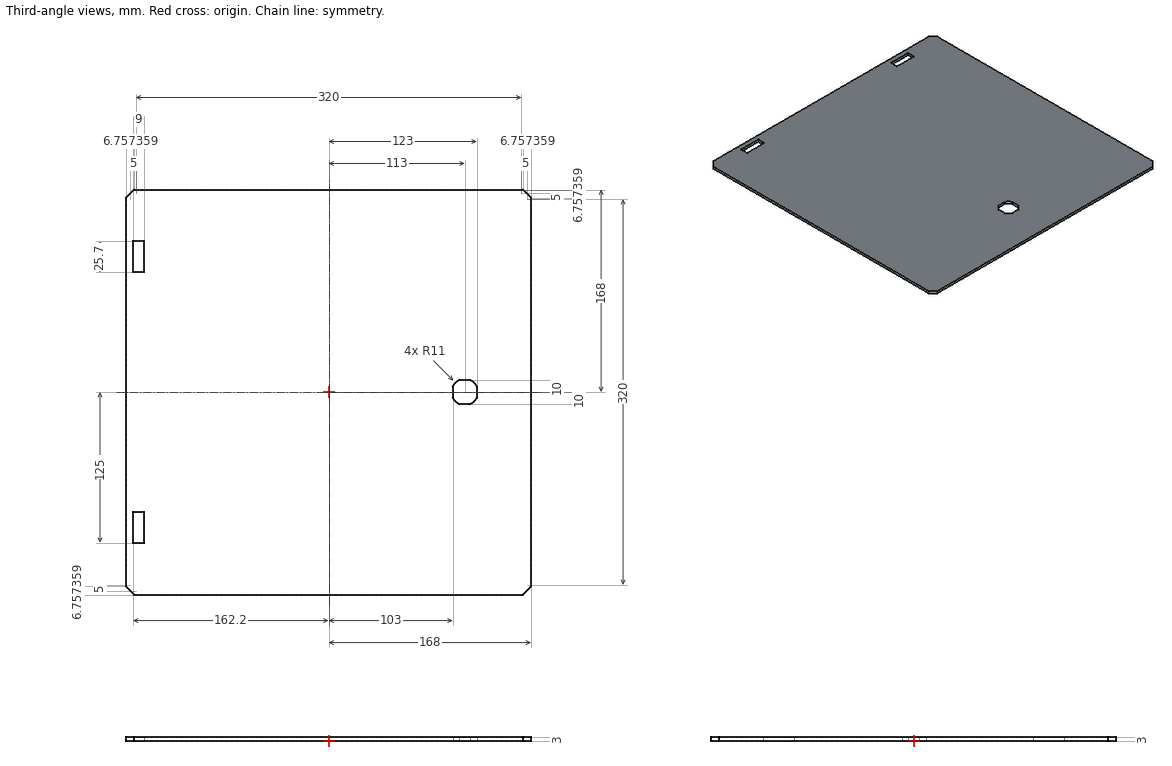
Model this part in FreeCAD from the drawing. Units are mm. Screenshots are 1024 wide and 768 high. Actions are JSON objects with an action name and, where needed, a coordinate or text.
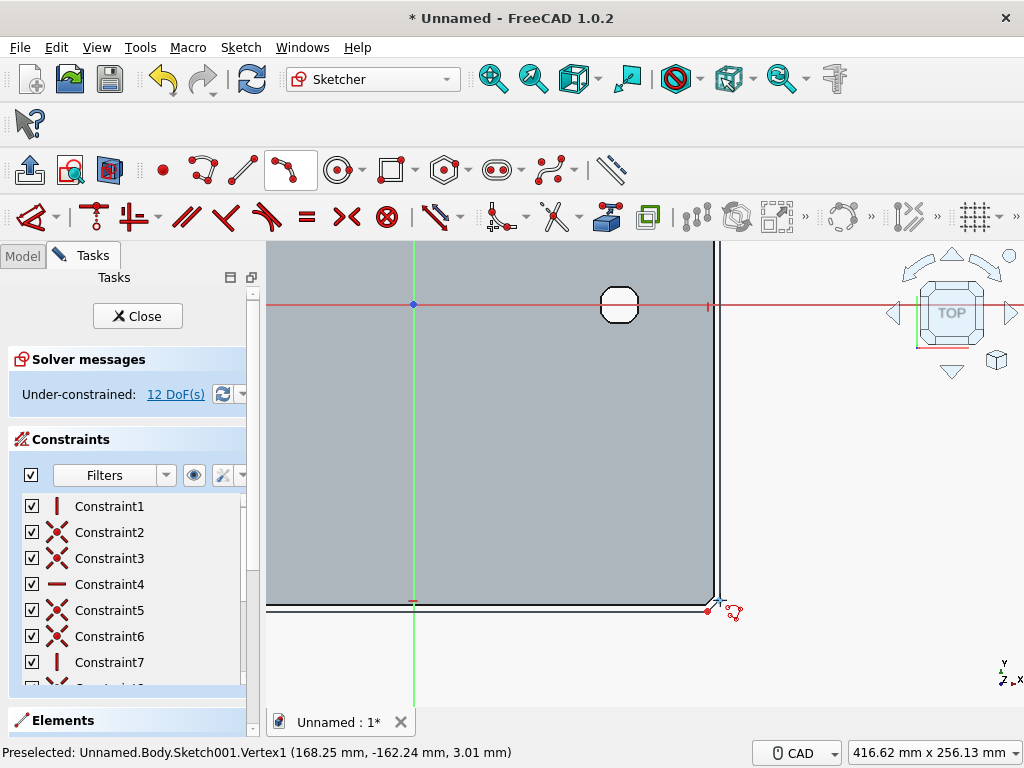
{"action": "scroll", "coordinate": [714, 596], "scroll_direction": "up", "scroll_amount": 6}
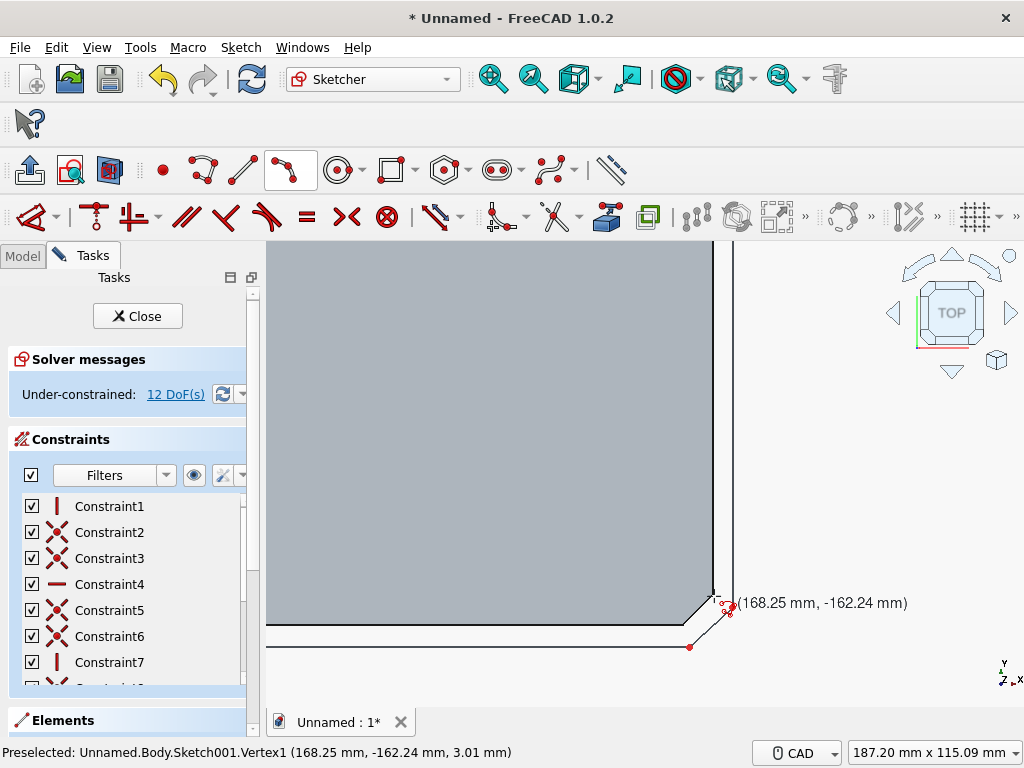
{"action": "left_click", "coordinate": [713, 594]}
{"action": "left_click", "coordinate": [683, 625]}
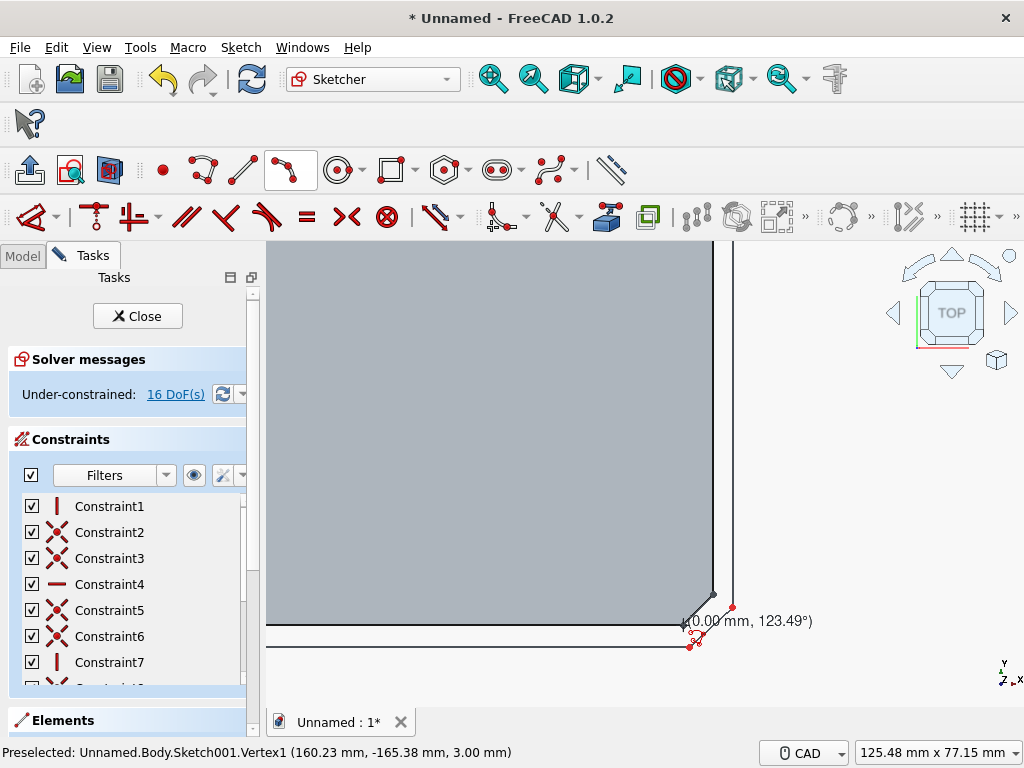
{"action": "scroll", "coordinate": [711, 606], "scroll_direction": "down", "scroll_amount": 10}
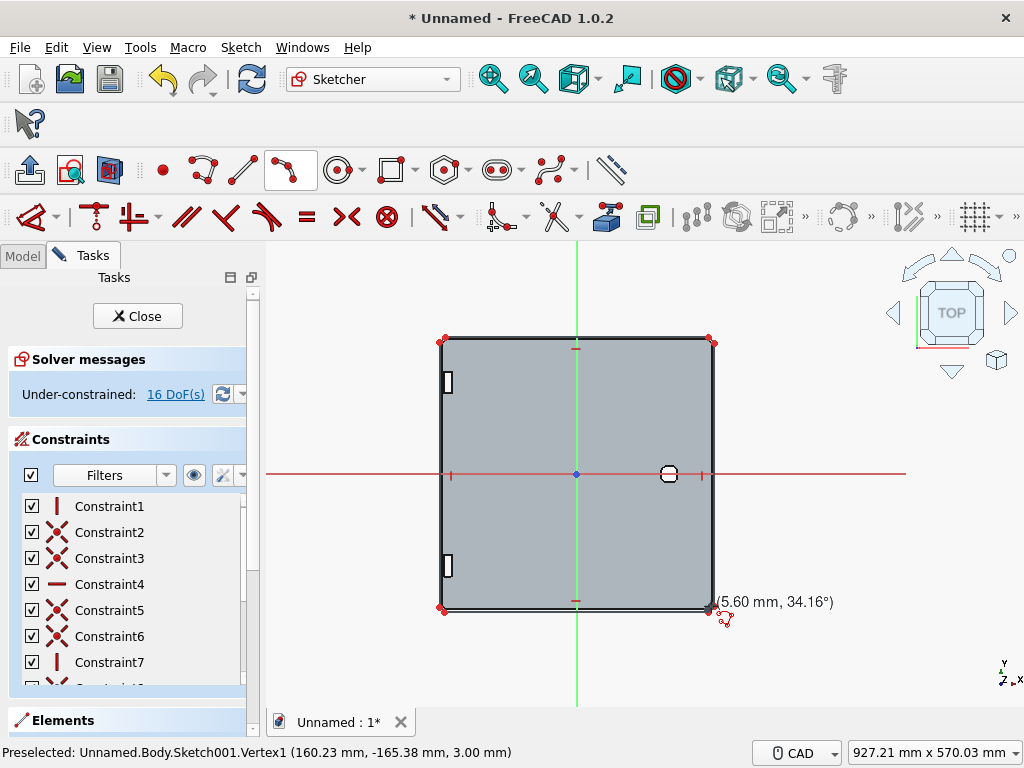
{"action": "scroll", "coordinate": [446, 609], "scroll_direction": "up", "scroll_amount": 10}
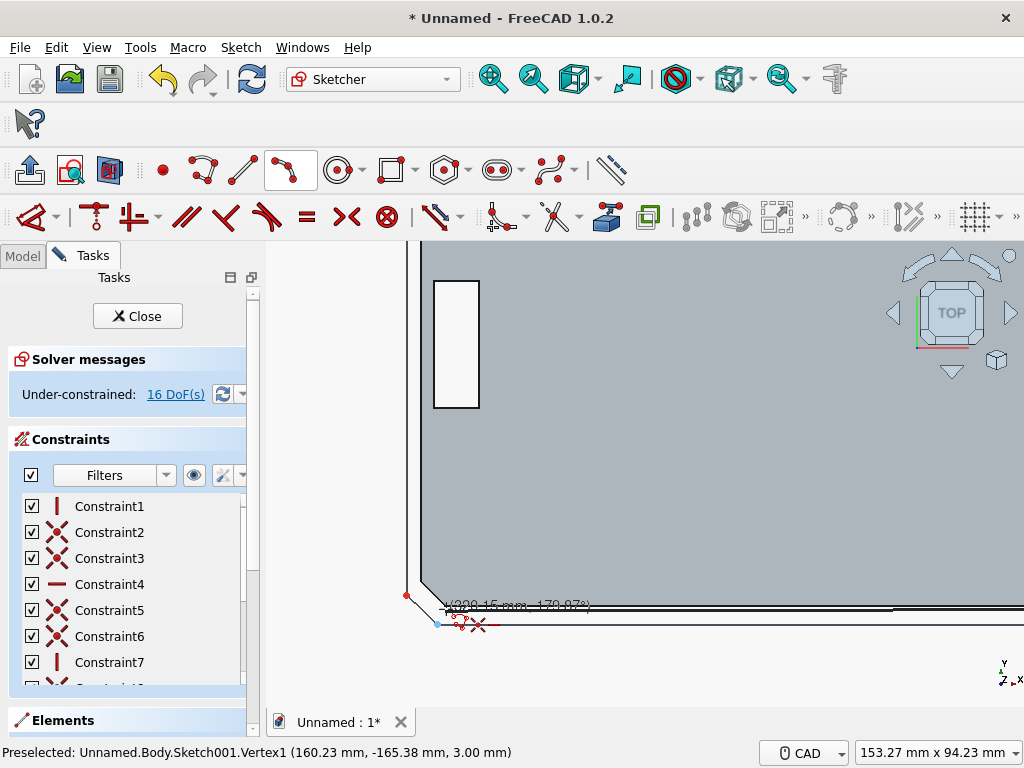
{"action": "left_click", "coordinate": [445, 606]}
{"action": "left_click", "coordinate": [415, 575]}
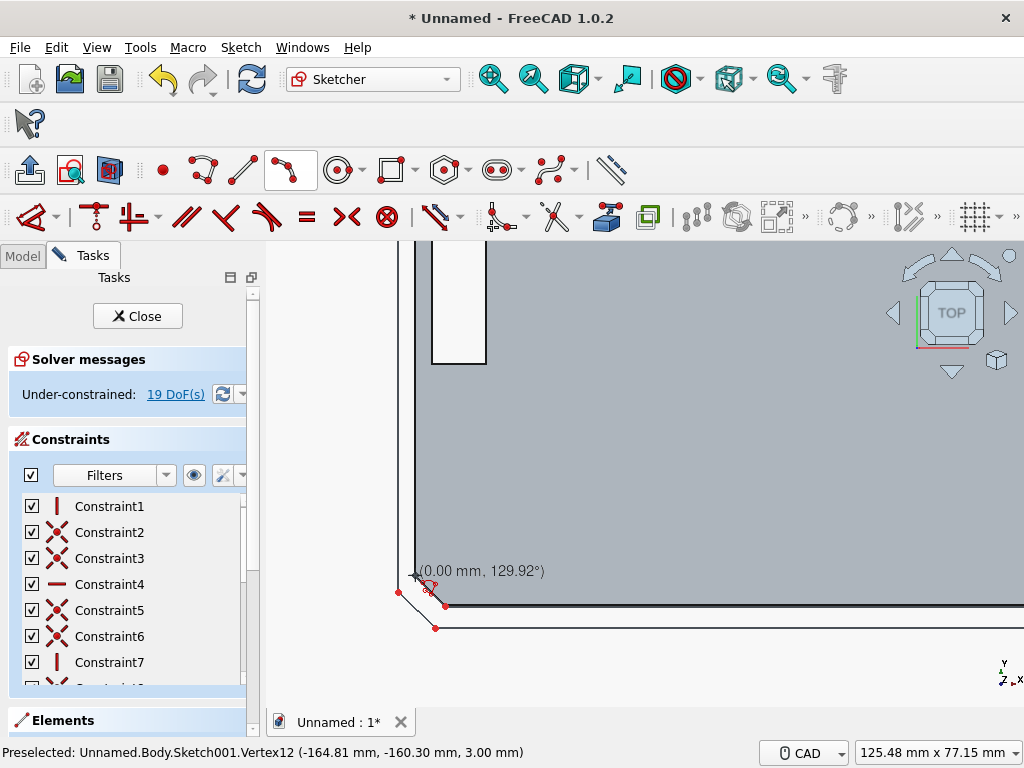
{"action": "scroll", "coordinate": [446, 609], "scroll_direction": "down", "scroll_amount": 10}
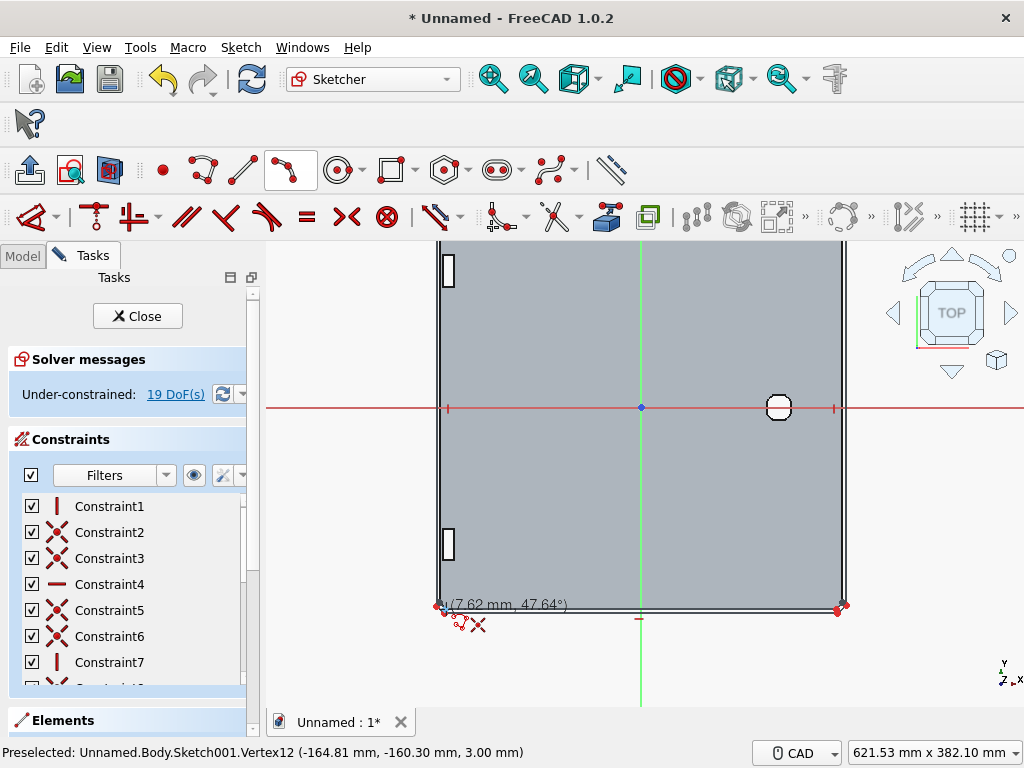
{"action": "scroll", "coordinate": [442, 344], "scroll_direction": "up", "scroll_amount": 10}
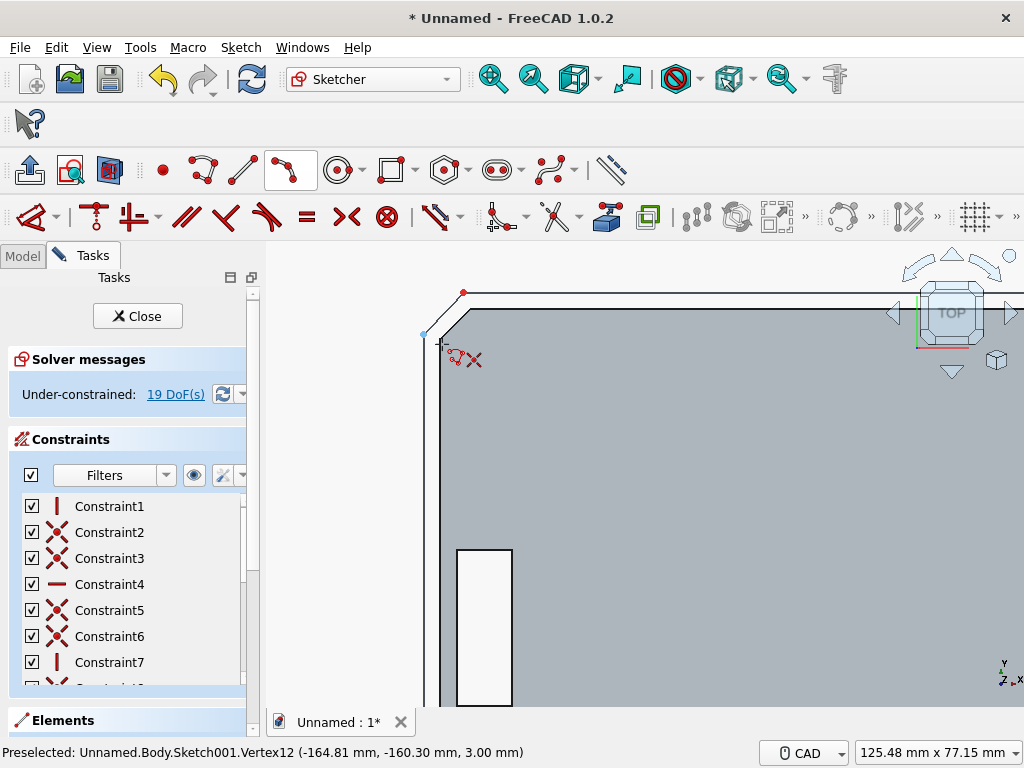
{"action": "left_click", "coordinate": [441, 339]}
{"action": "left_click", "coordinate": [471, 309]}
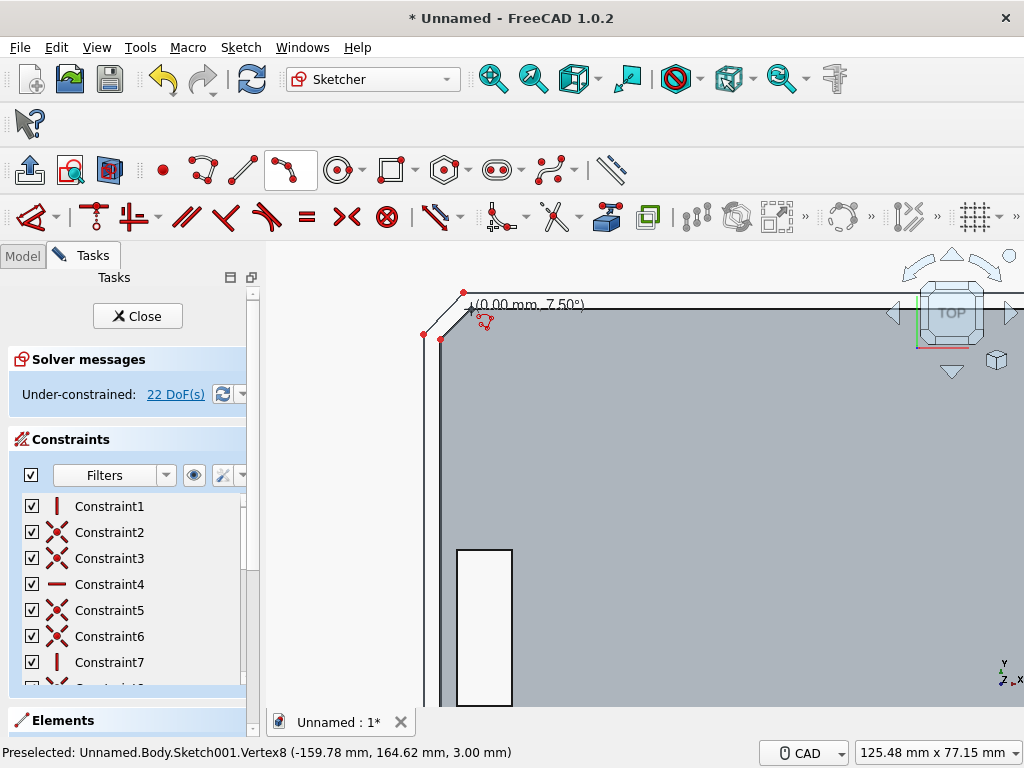
{"action": "scroll", "coordinate": [442, 344], "scroll_direction": "down", "scroll_amount": 10}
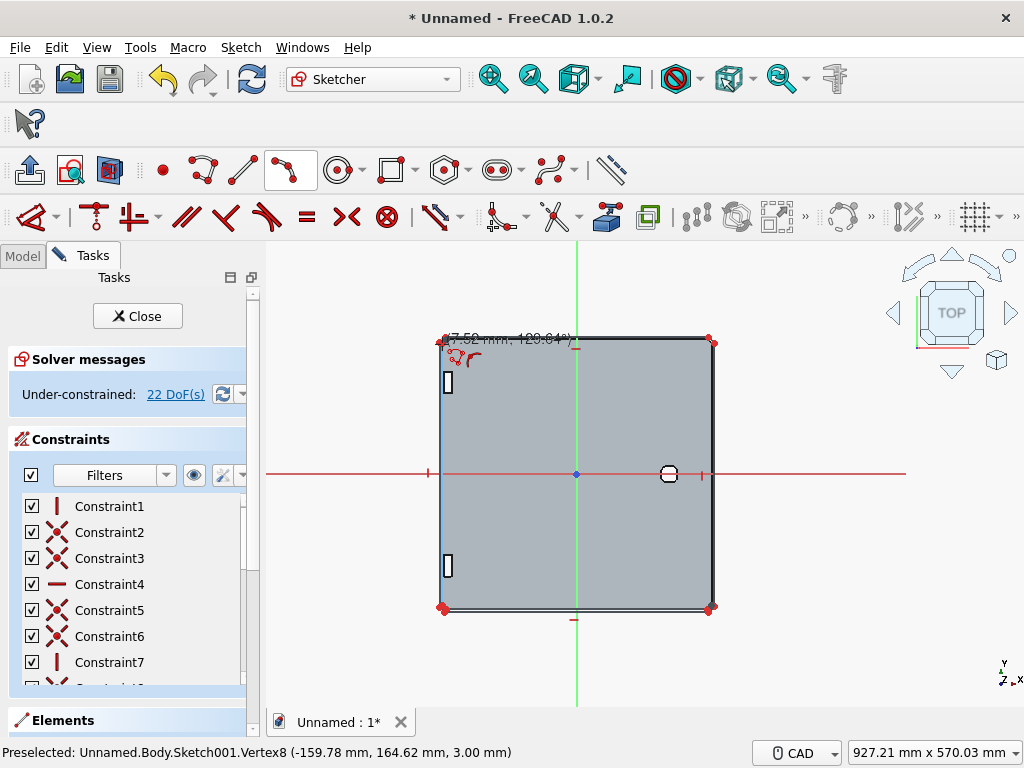
{"action": "scroll", "coordinate": [708, 339], "scroll_direction": "up", "scroll_amount": 10}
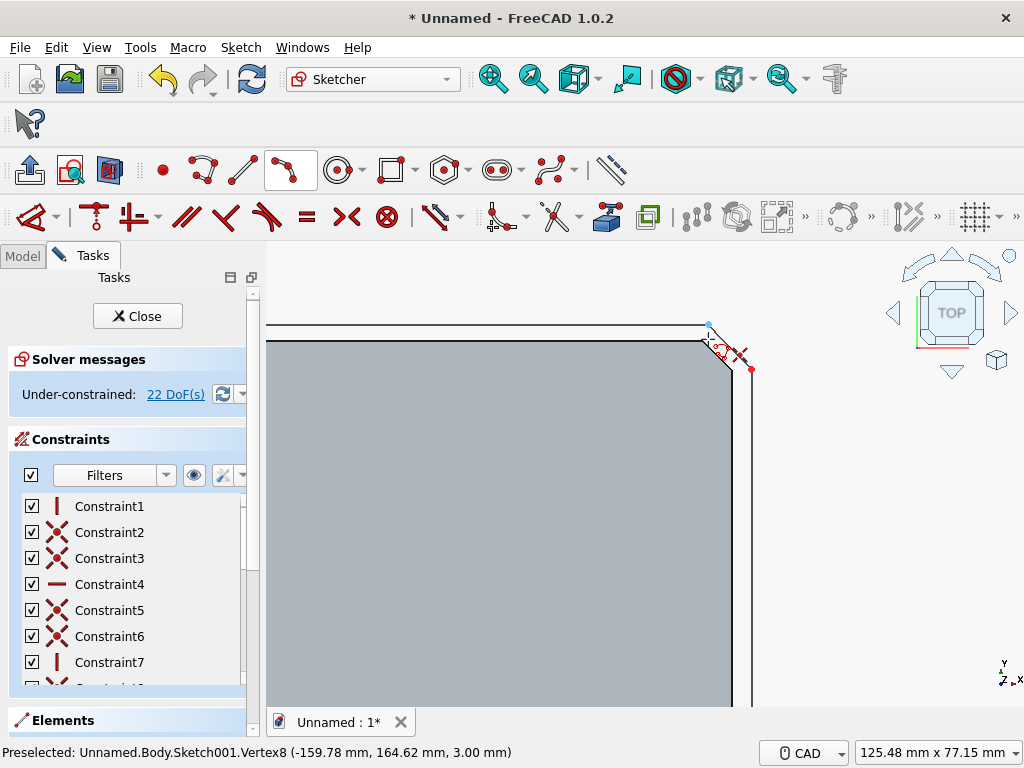
{"action": "left_click", "coordinate": [702, 341]}
{"action": "left_click", "coordinate": [732, 371]}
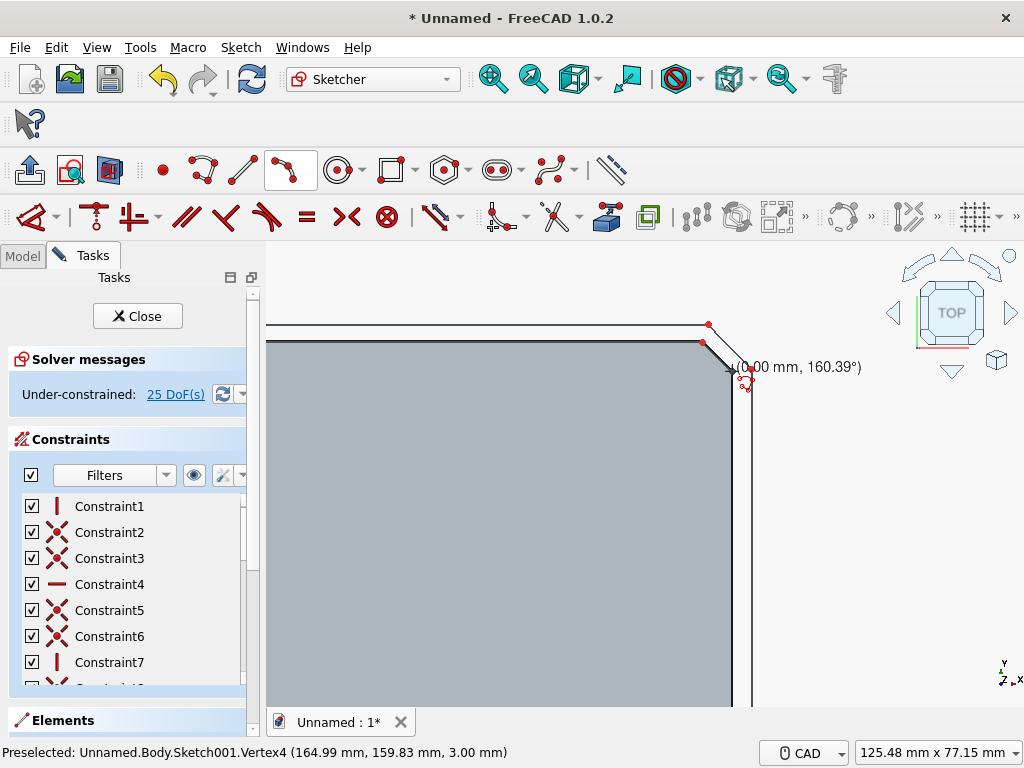
{"action": "scroll", "coordinate": [708, 339], "scroll_direction": "down", "scroll_amount": 10}